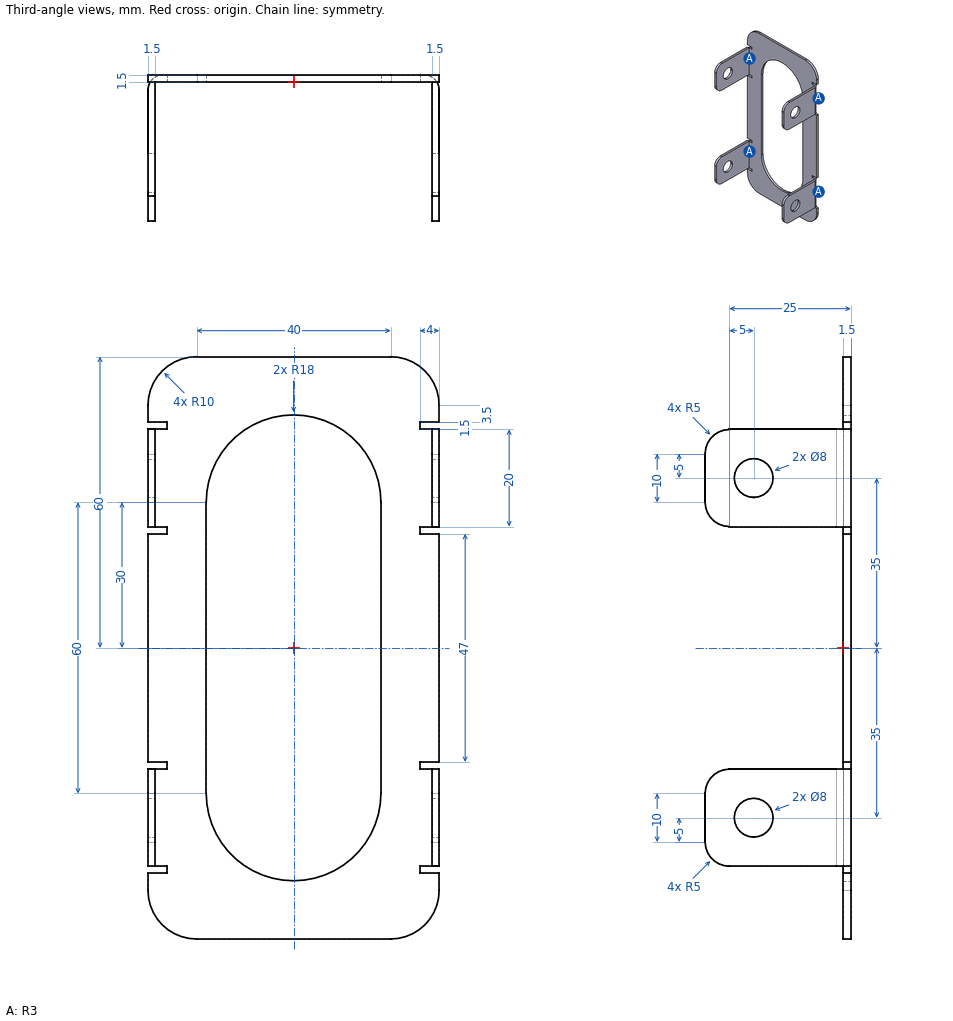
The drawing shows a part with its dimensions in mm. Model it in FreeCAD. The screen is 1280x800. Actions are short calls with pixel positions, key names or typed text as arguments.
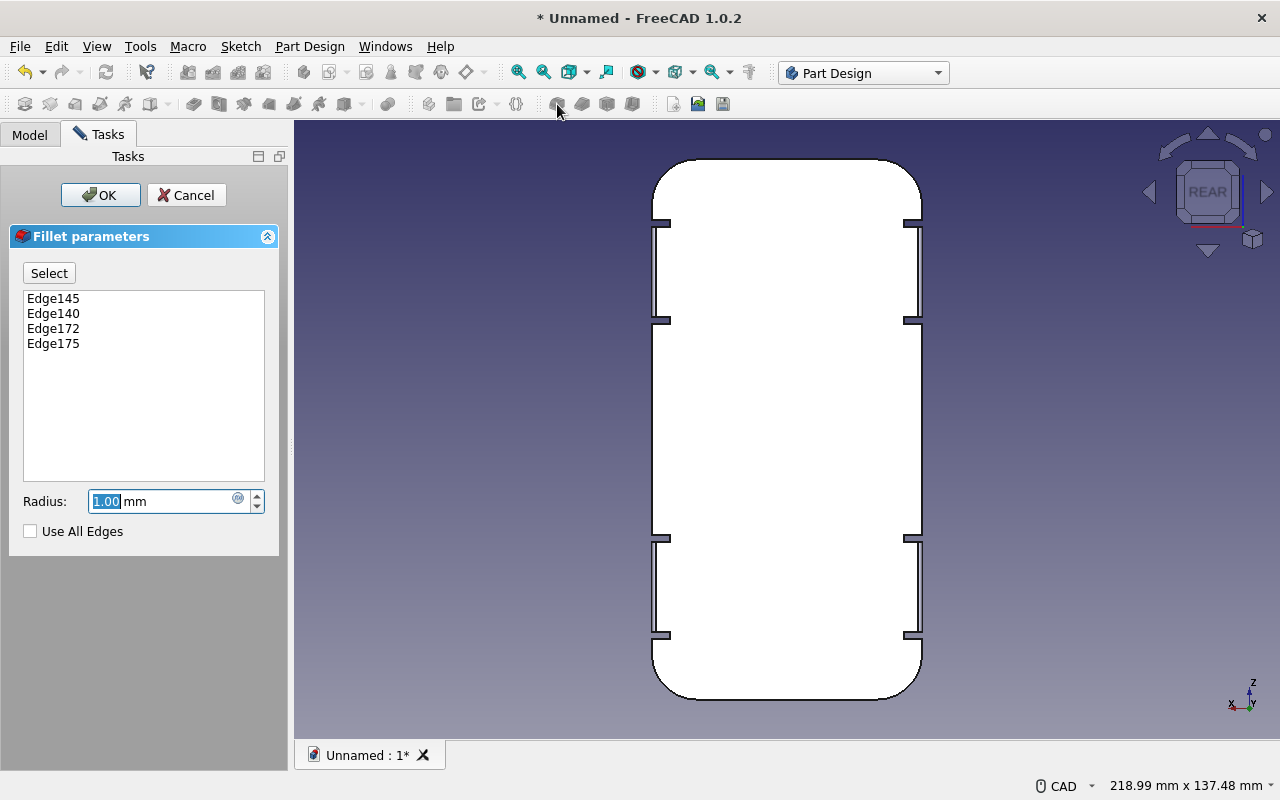
text(3)
key(Tab)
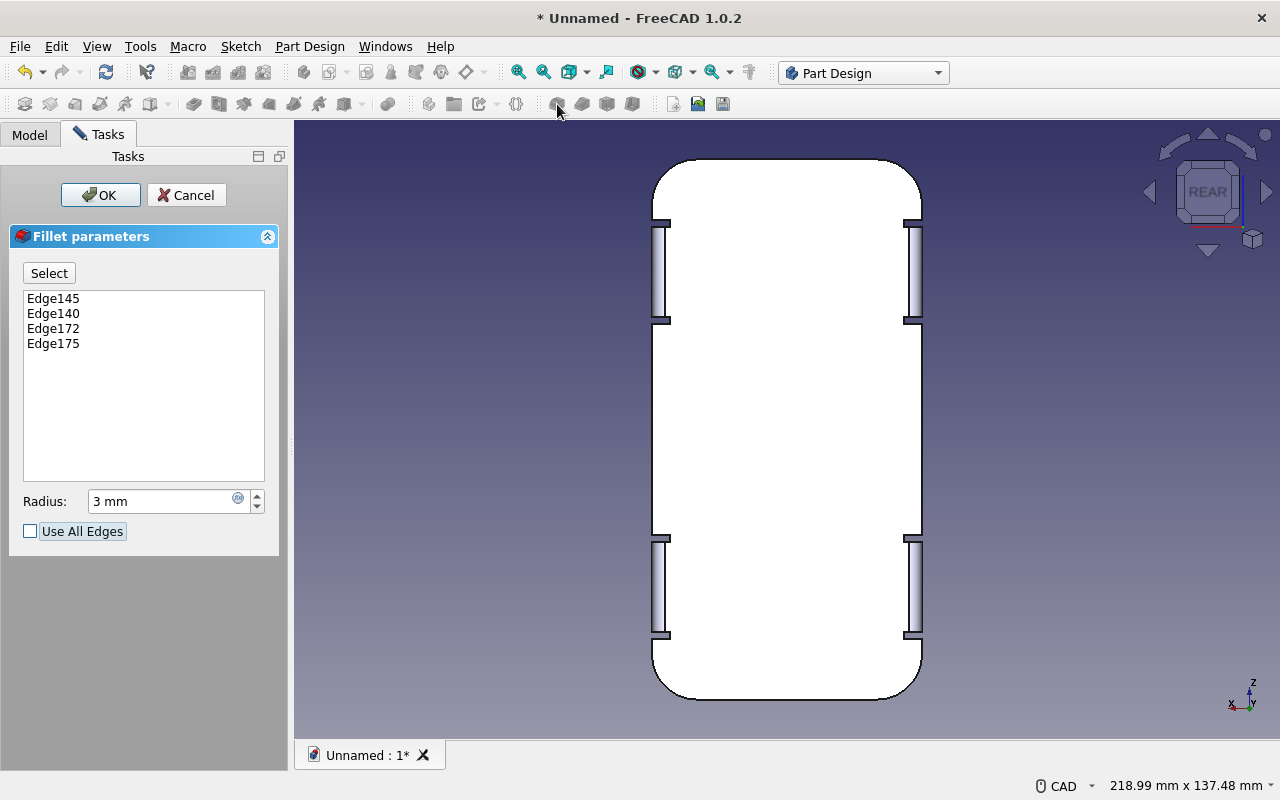
click(101, 195)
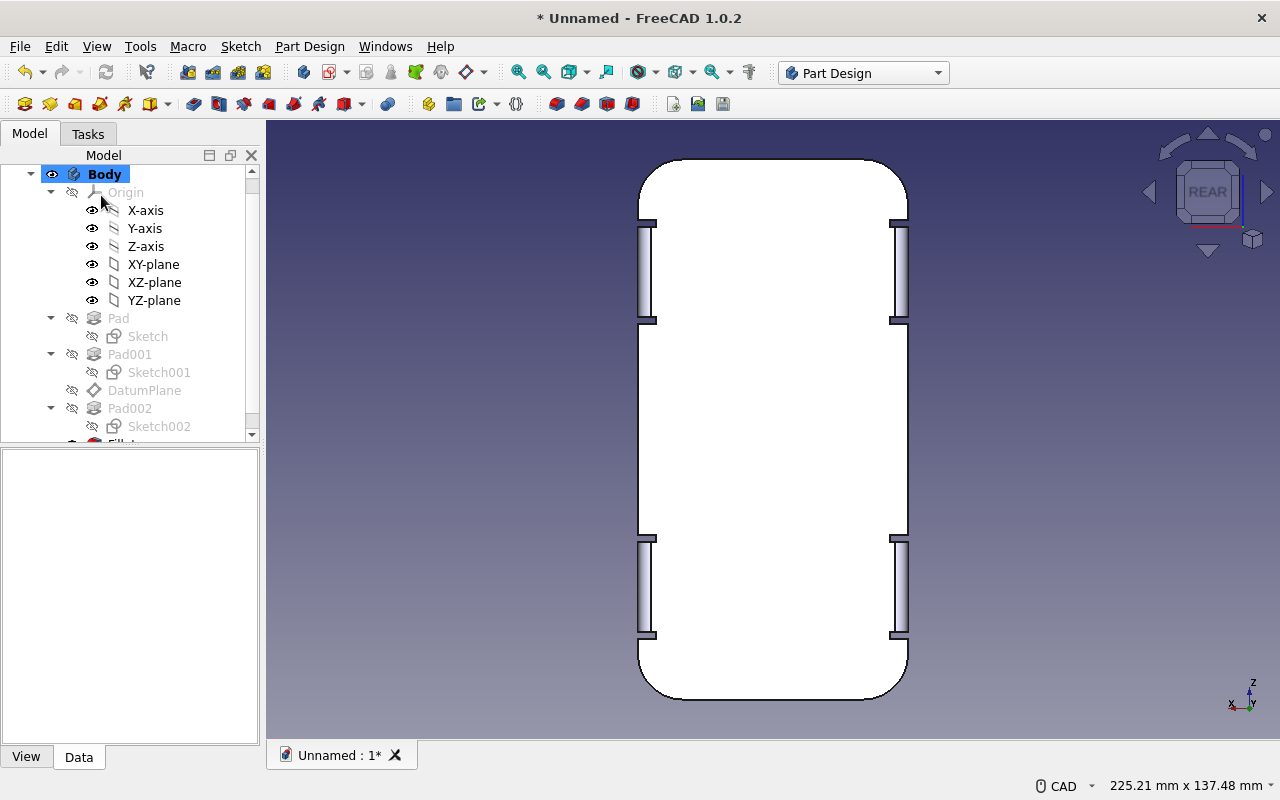
click(773, 429)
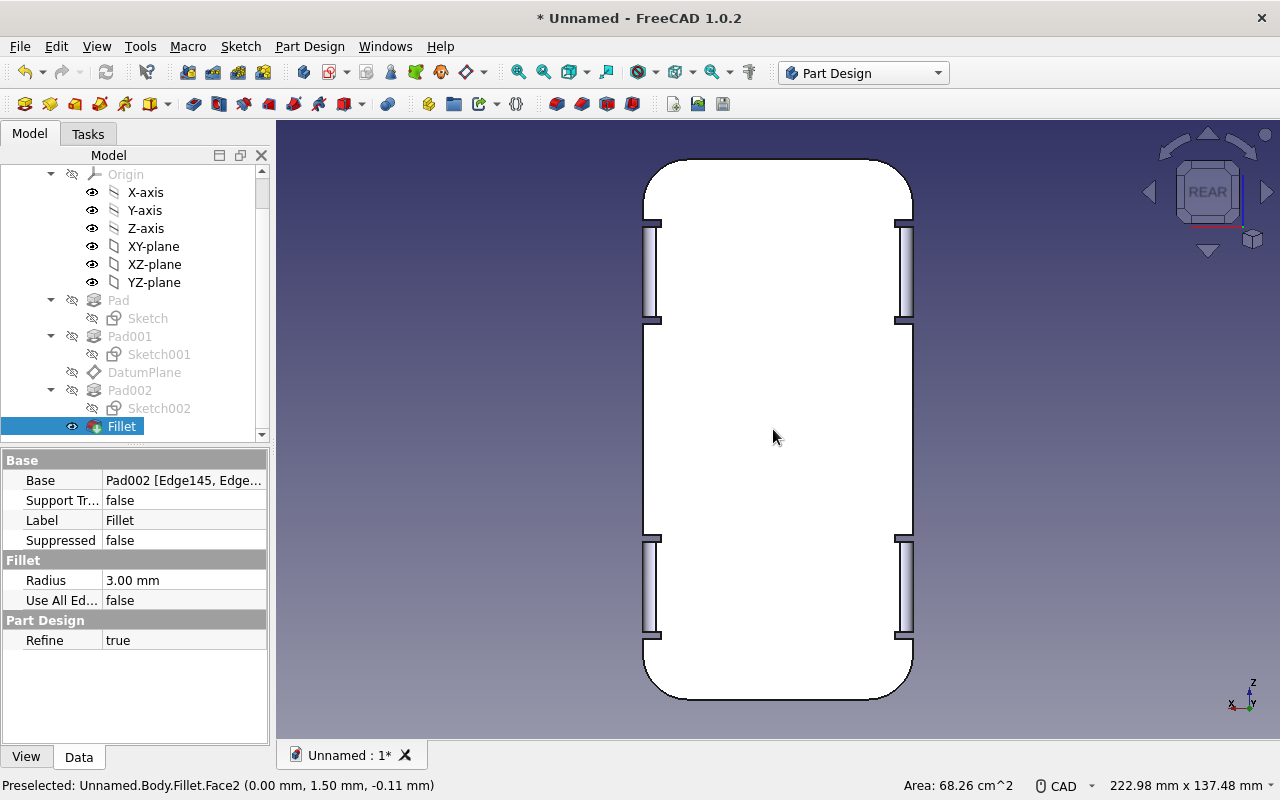
click(328, 72)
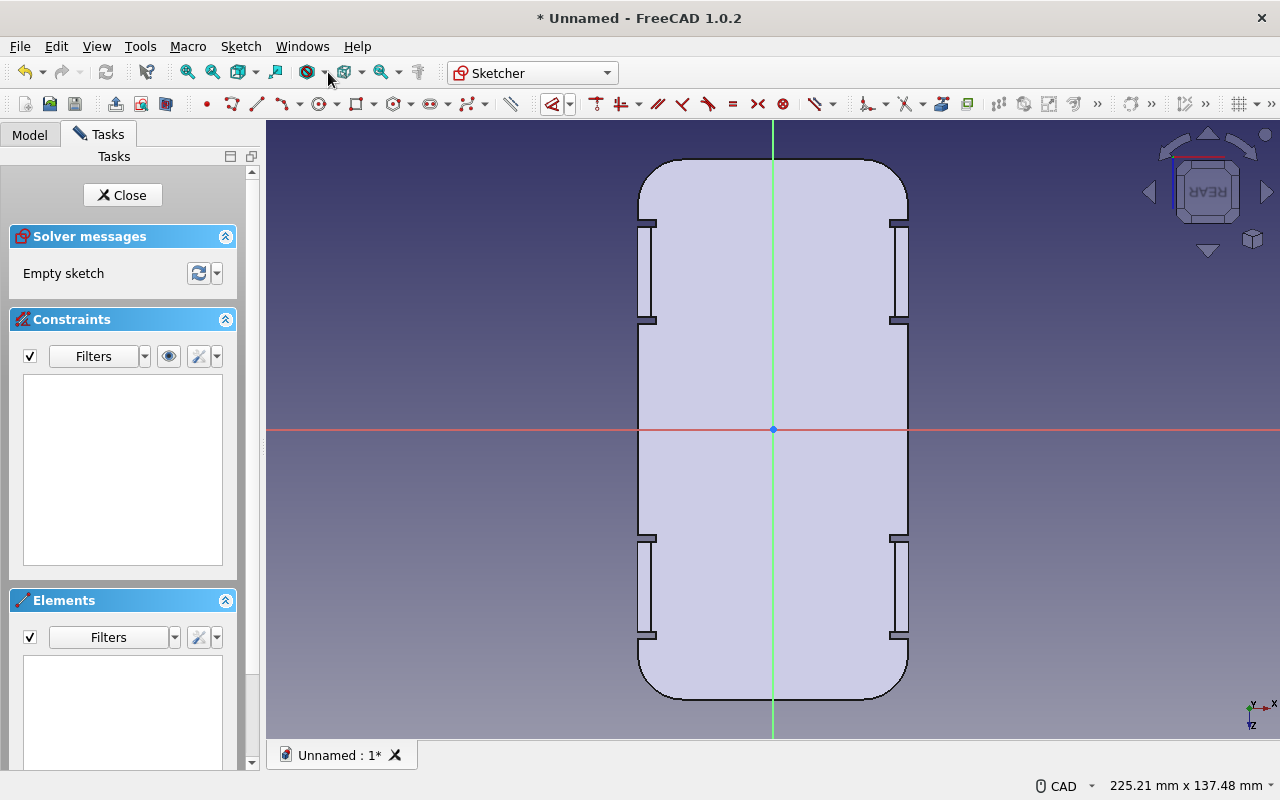
click(430, 104)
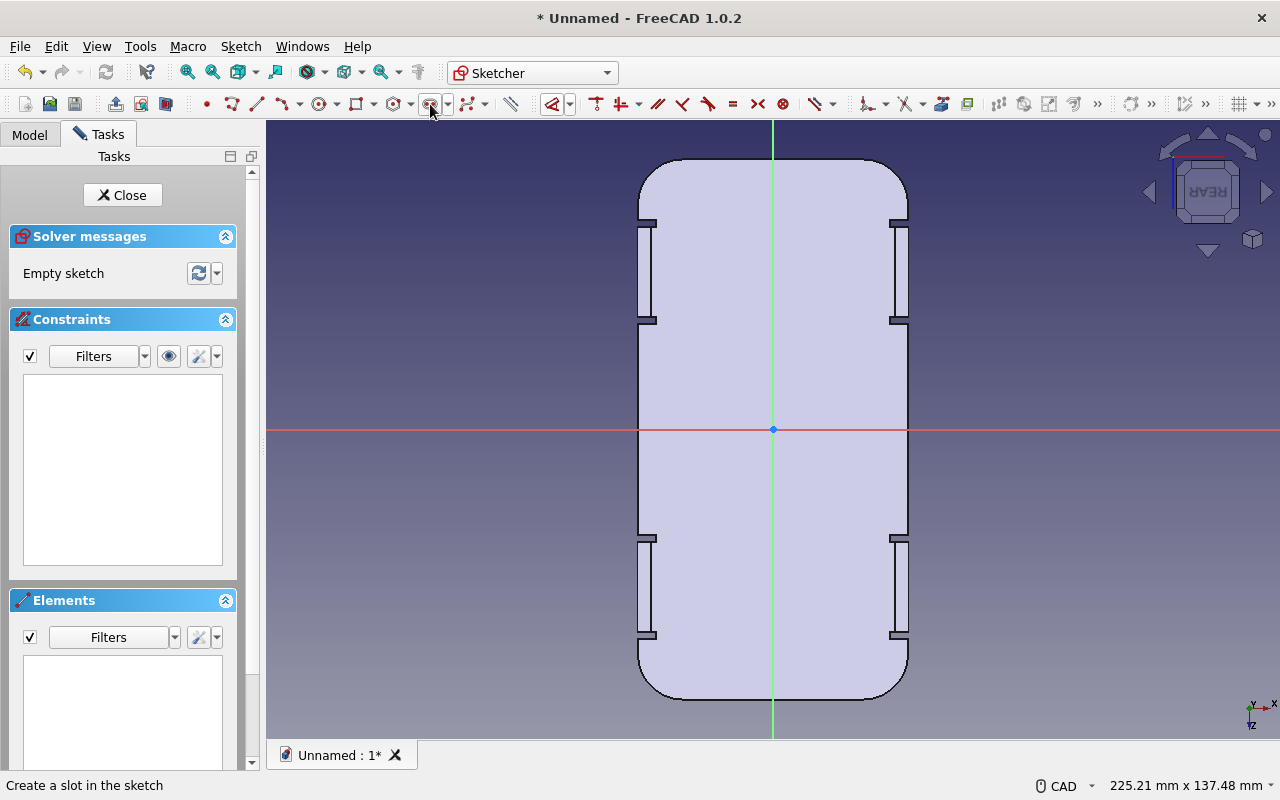
click(773, 565)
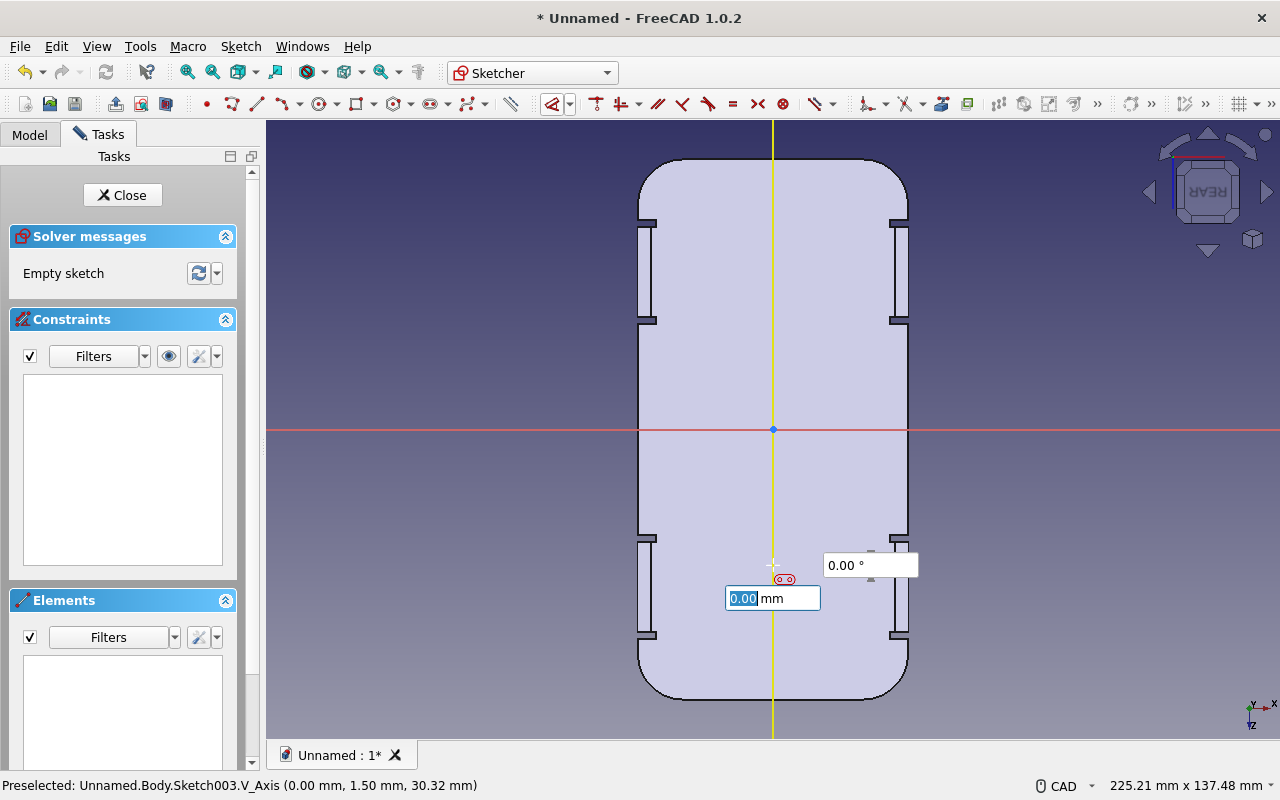
click(782, 294)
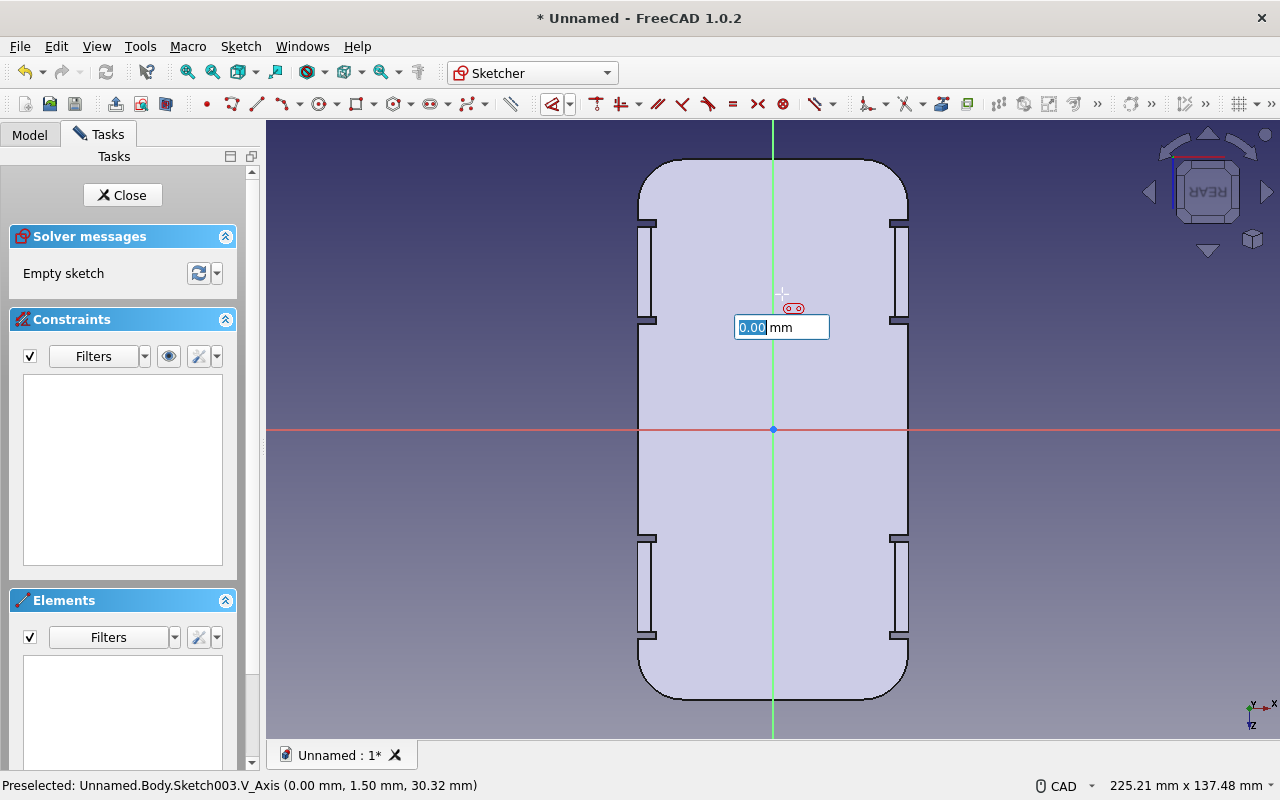
click(692, 389)
key(Escape)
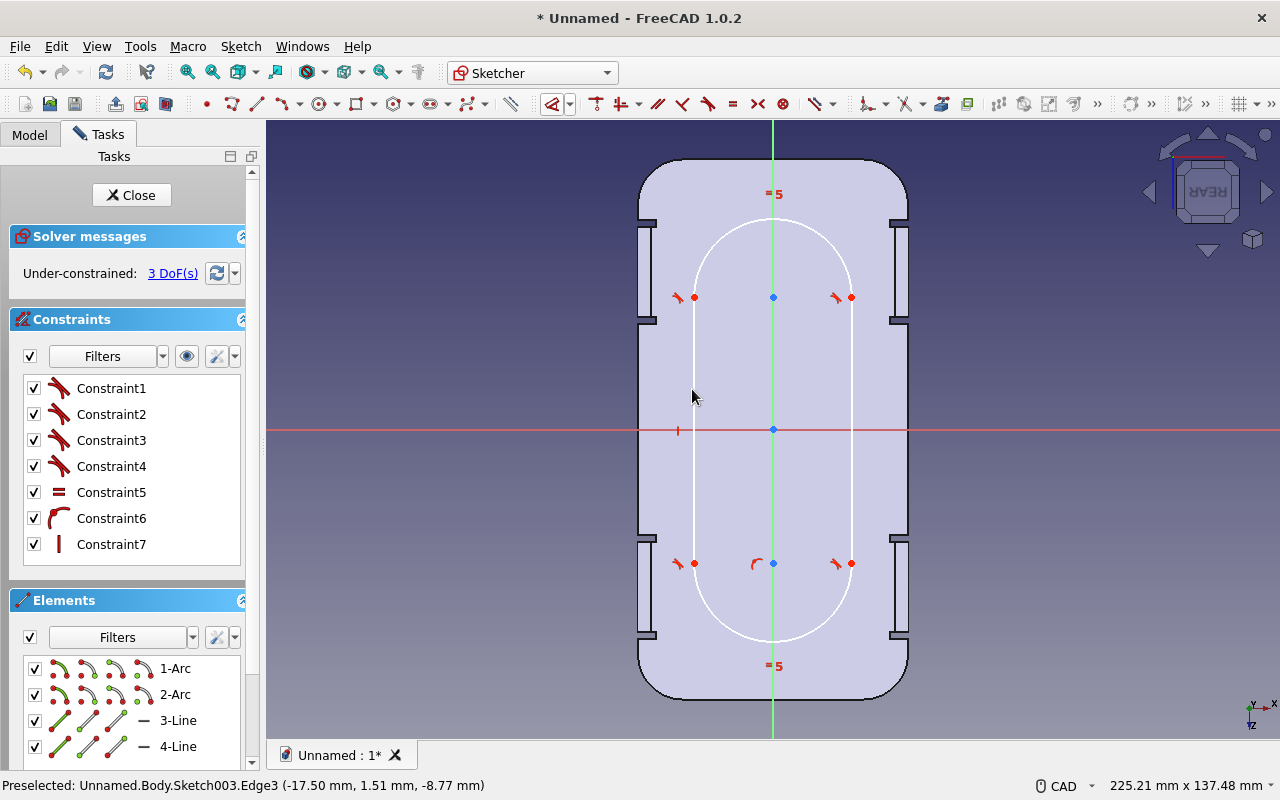
click(727, 627)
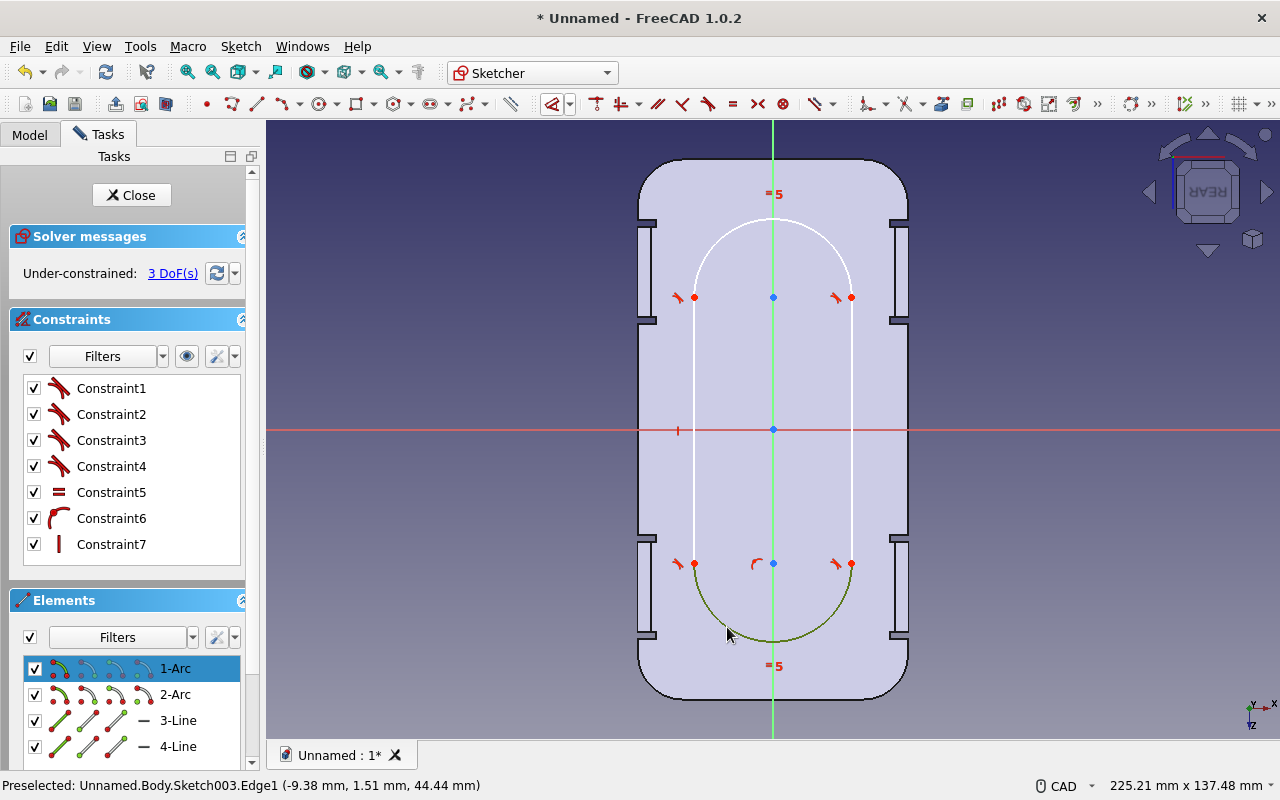
key(k)
key(r)